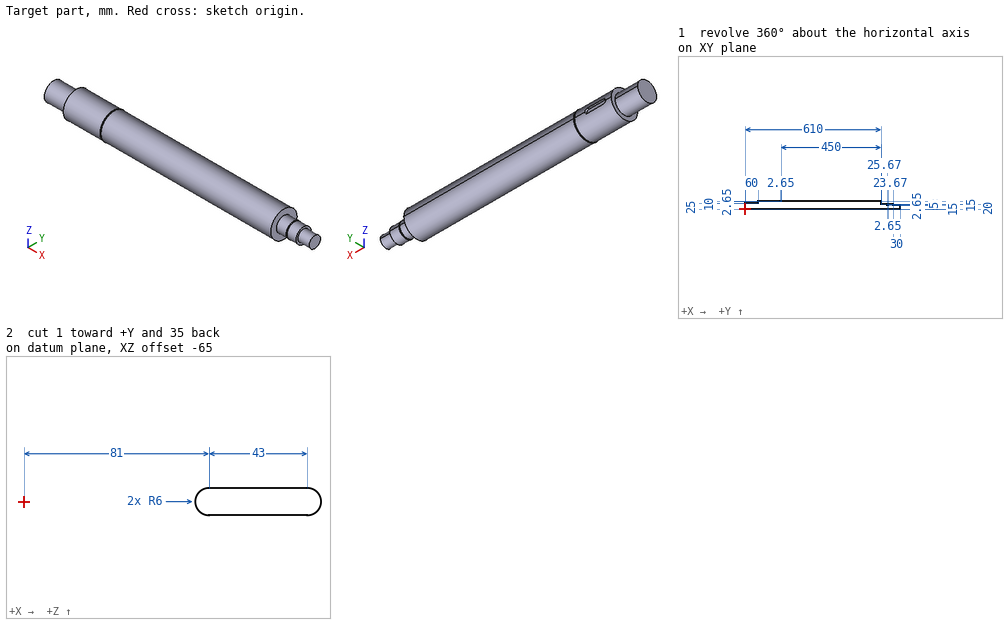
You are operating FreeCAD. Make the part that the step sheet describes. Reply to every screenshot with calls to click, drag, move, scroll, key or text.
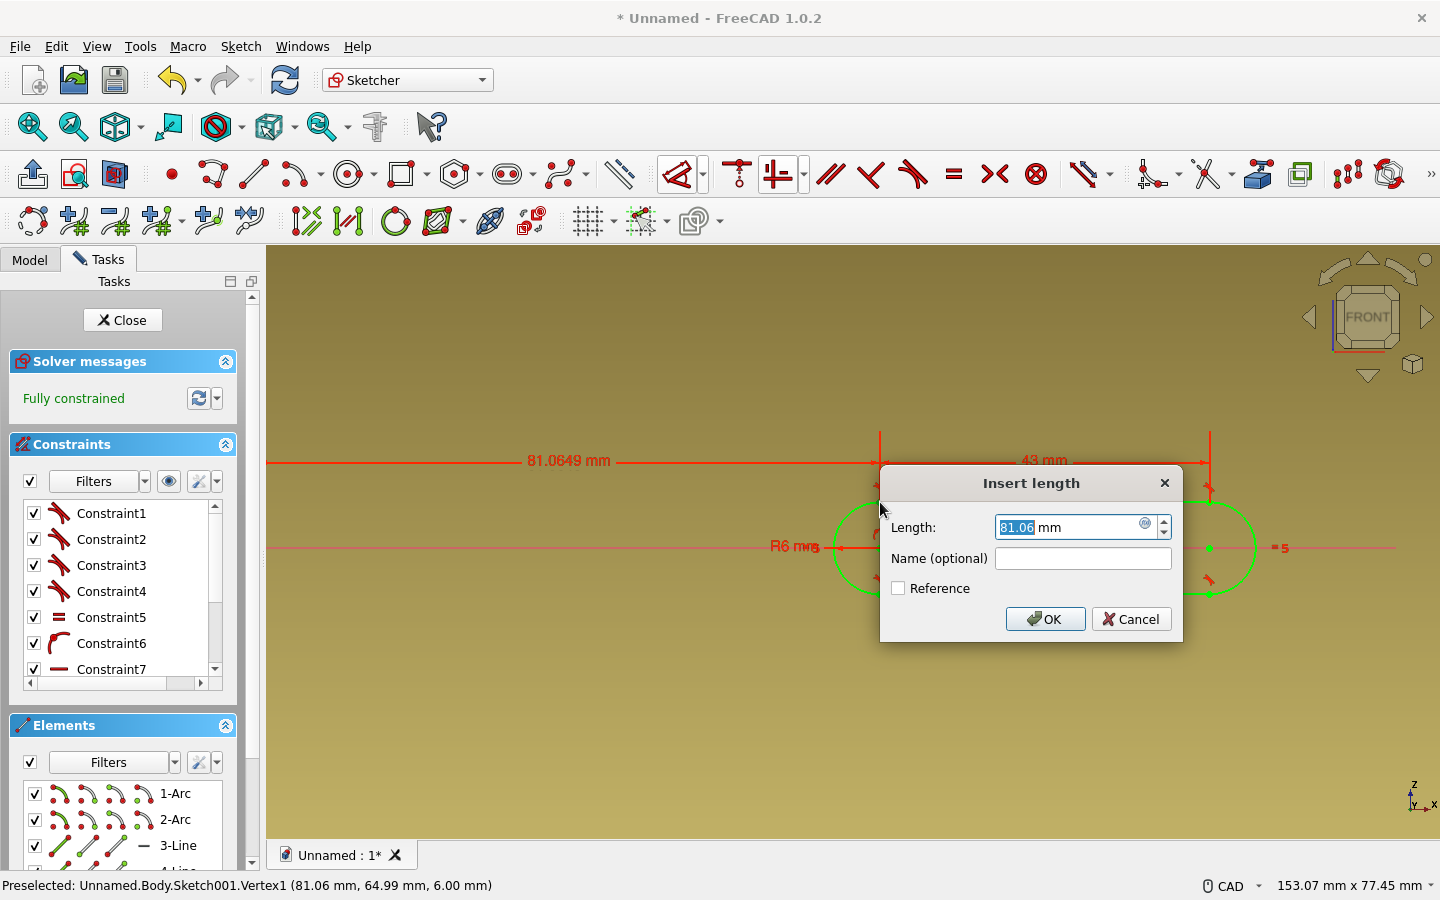
text(81)
key(Return)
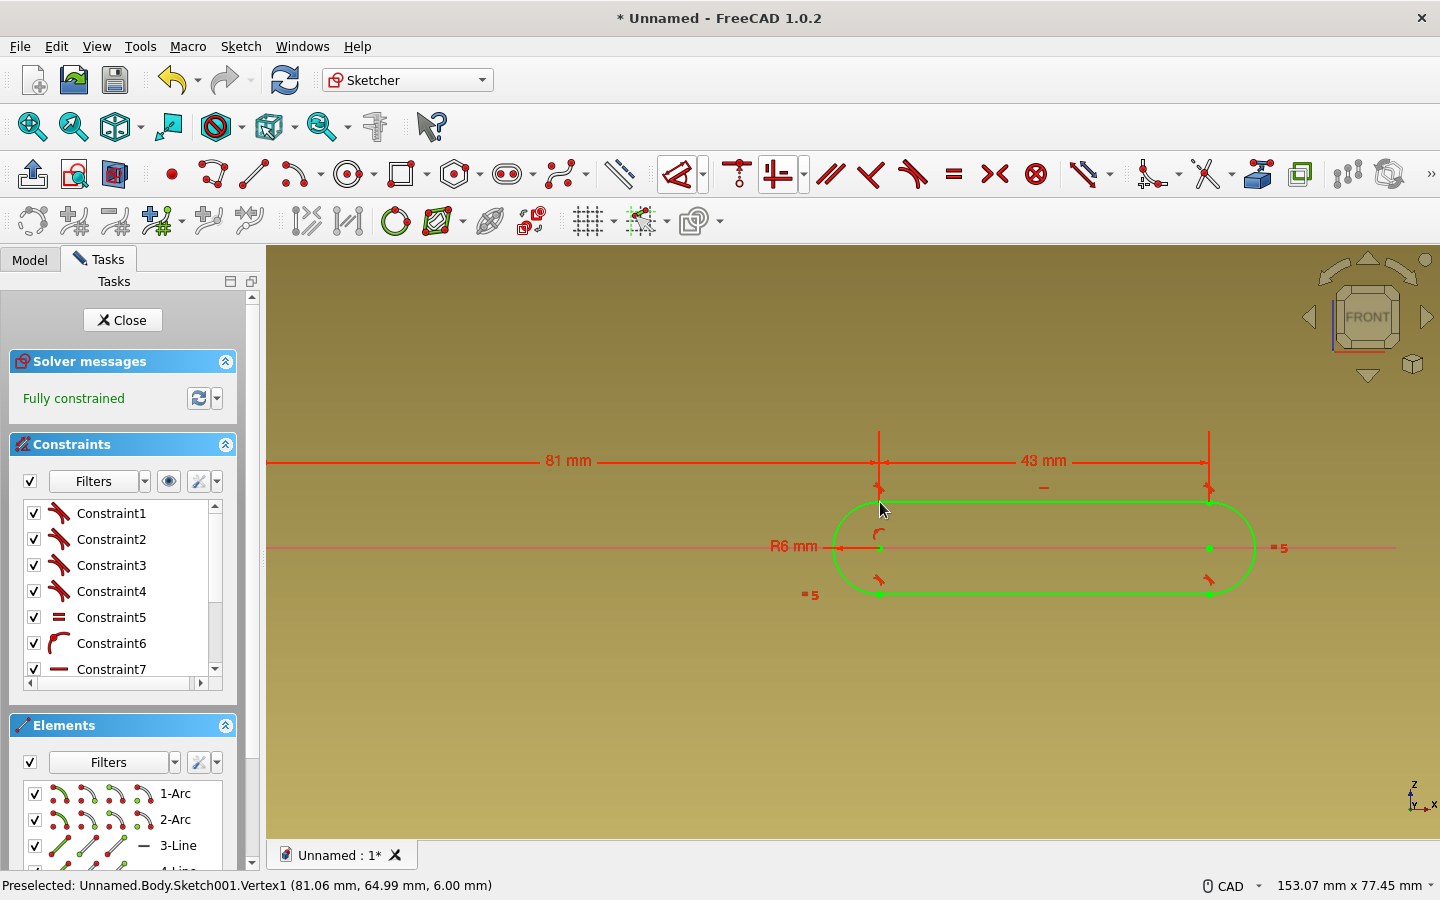
click(123, 320)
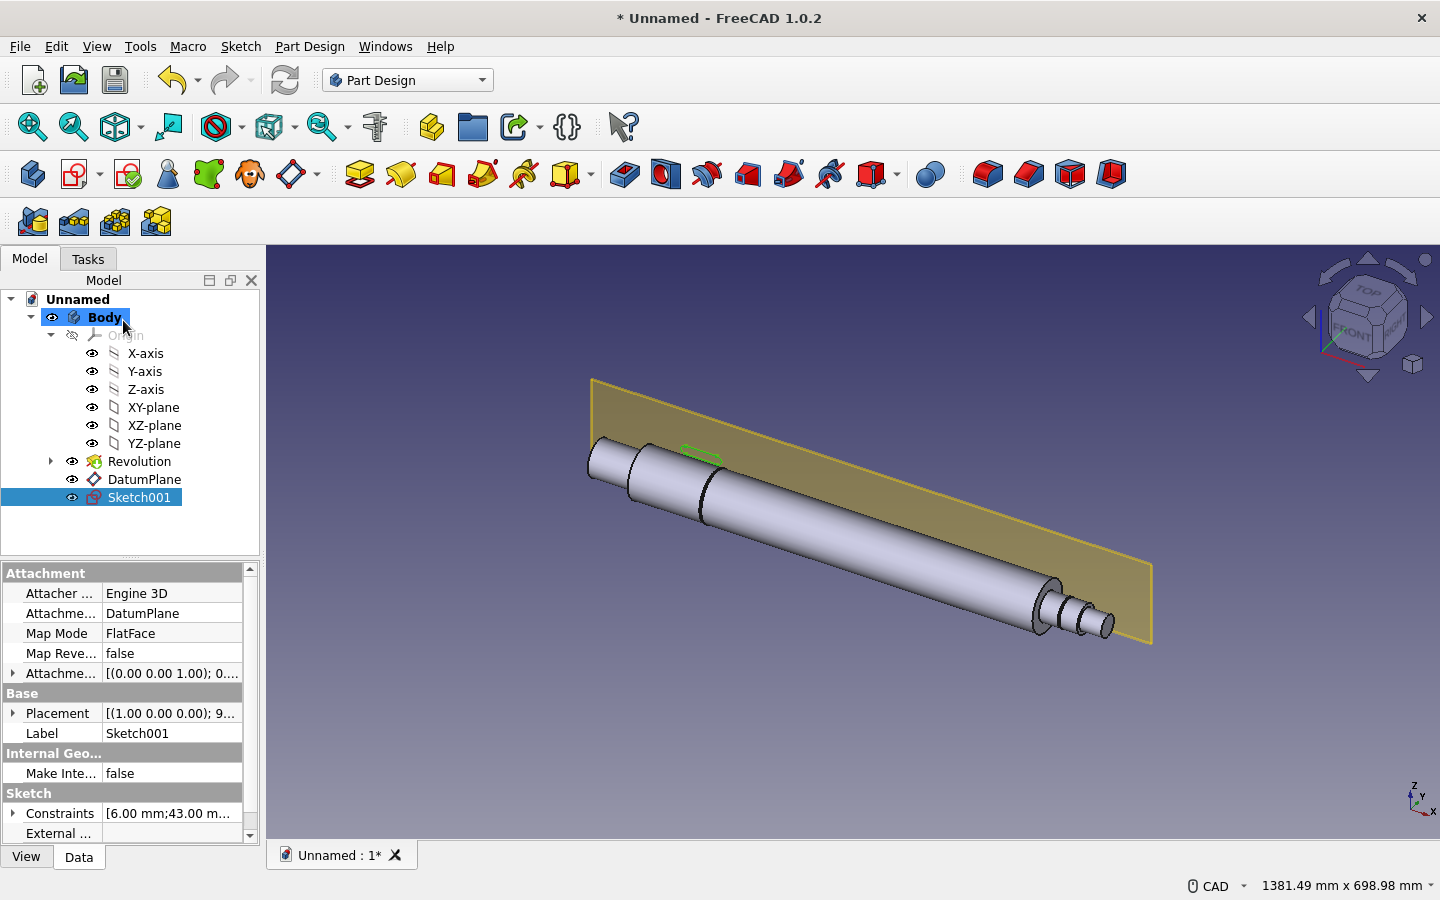
click(625, 174)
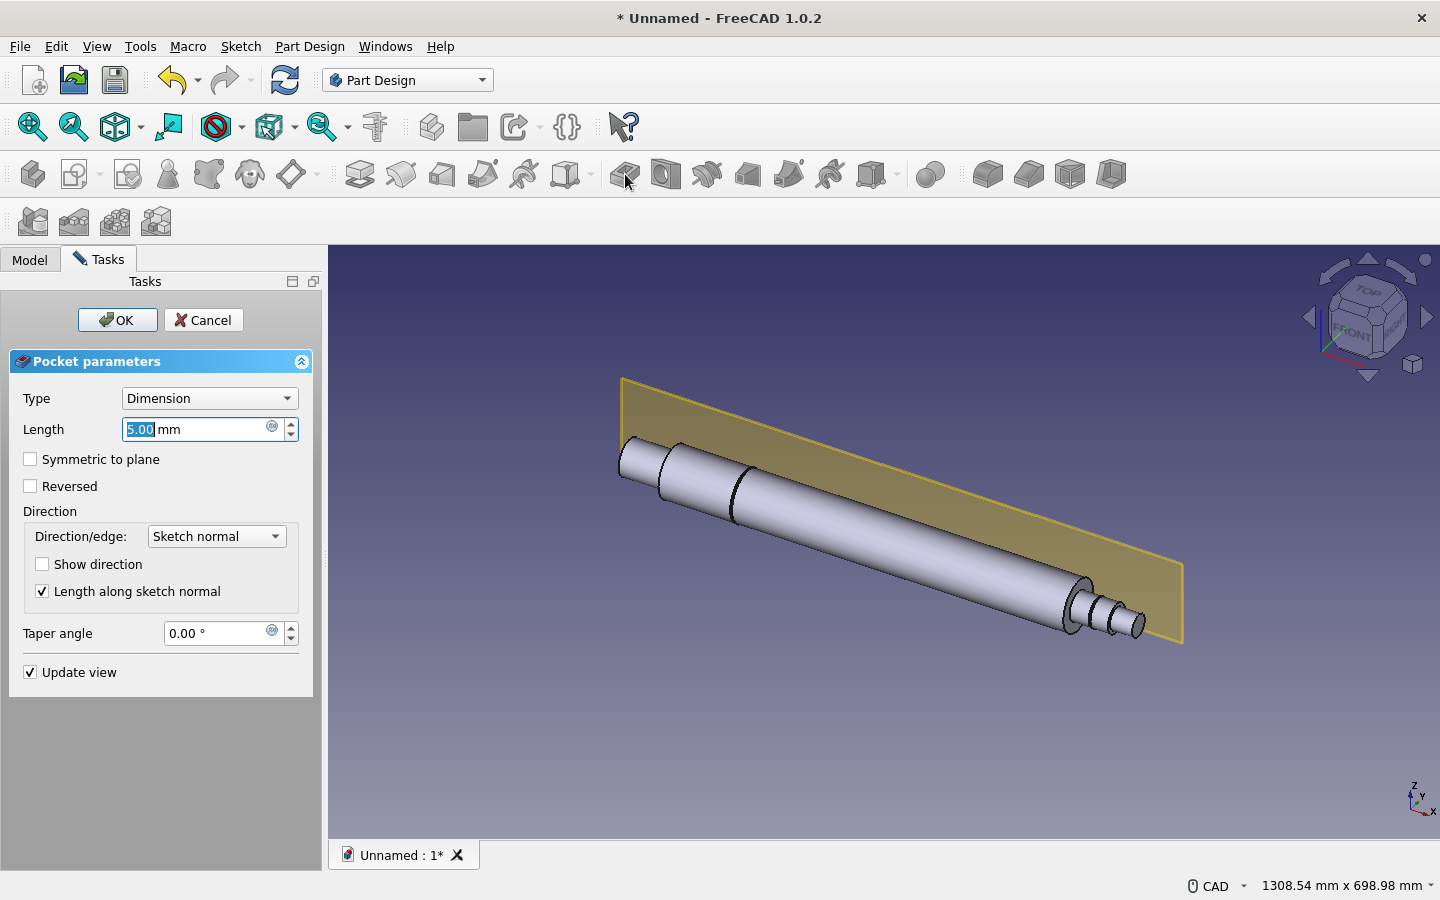
click(210, 398)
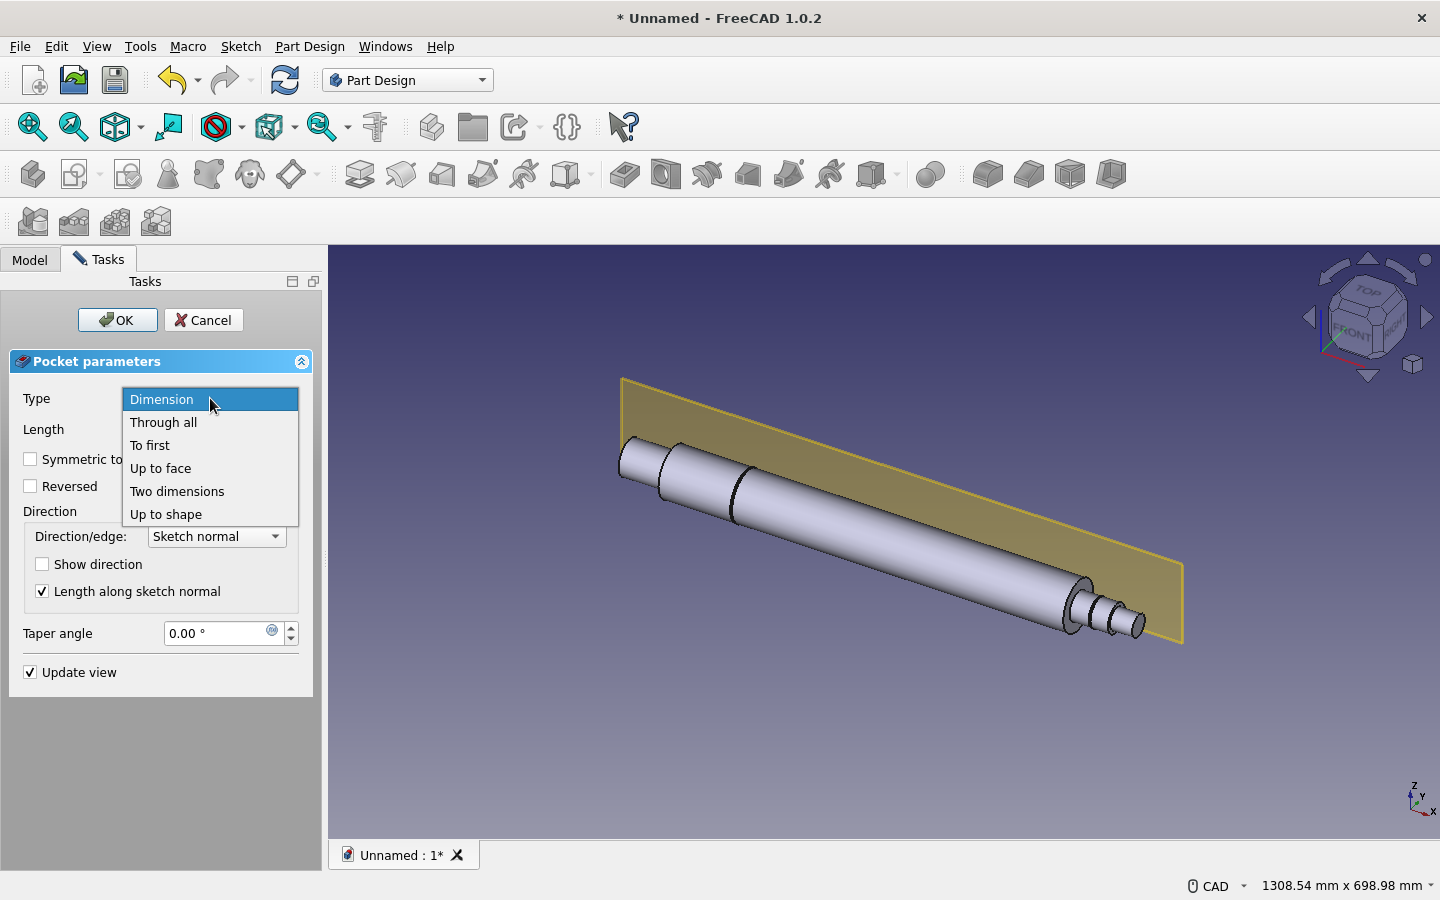
click(208, 492)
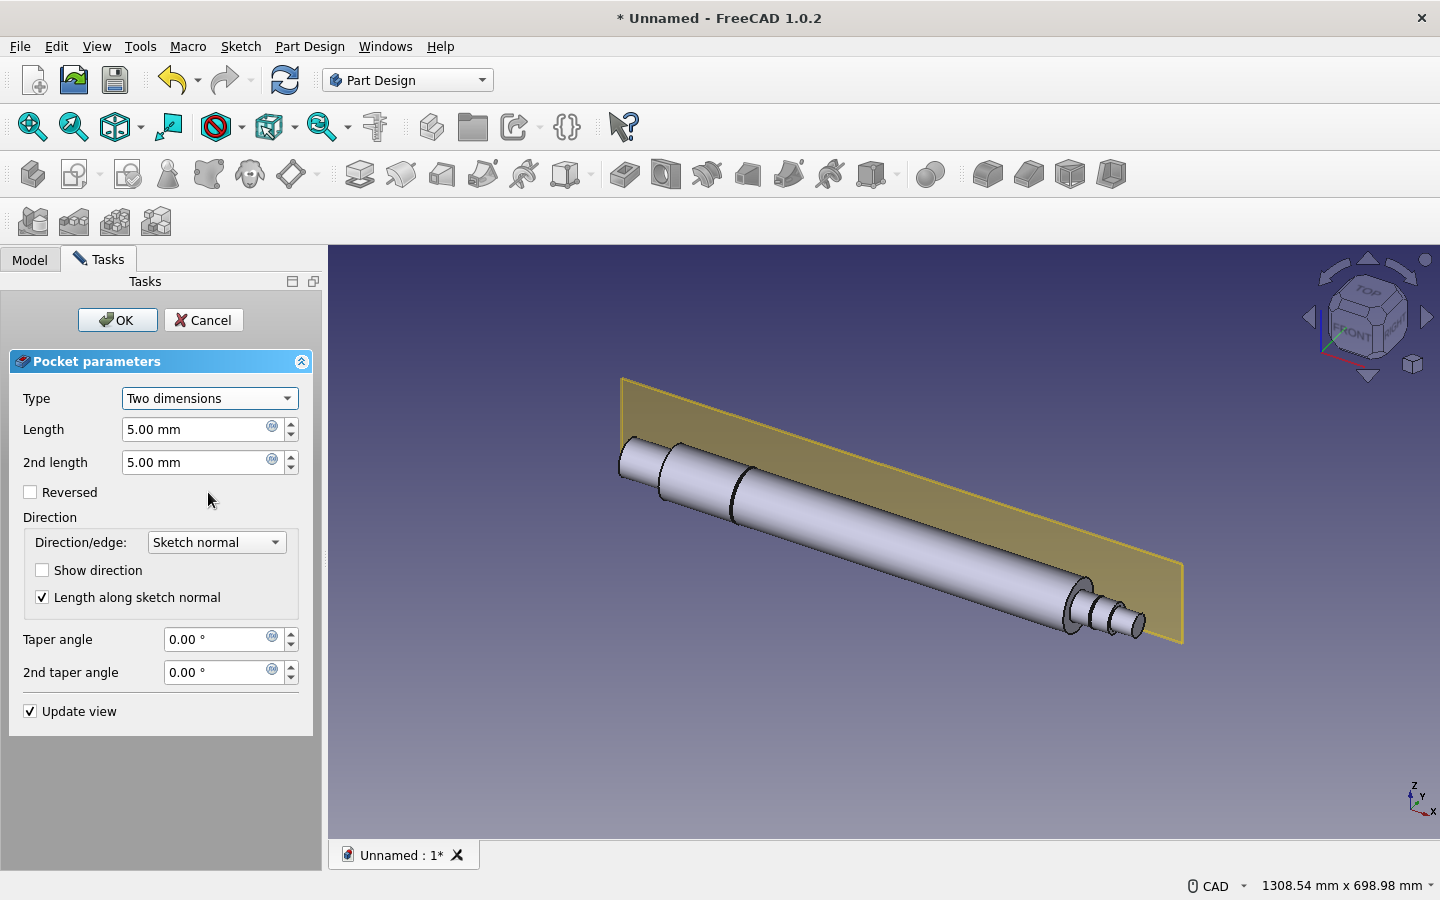
triple_click(204, 430)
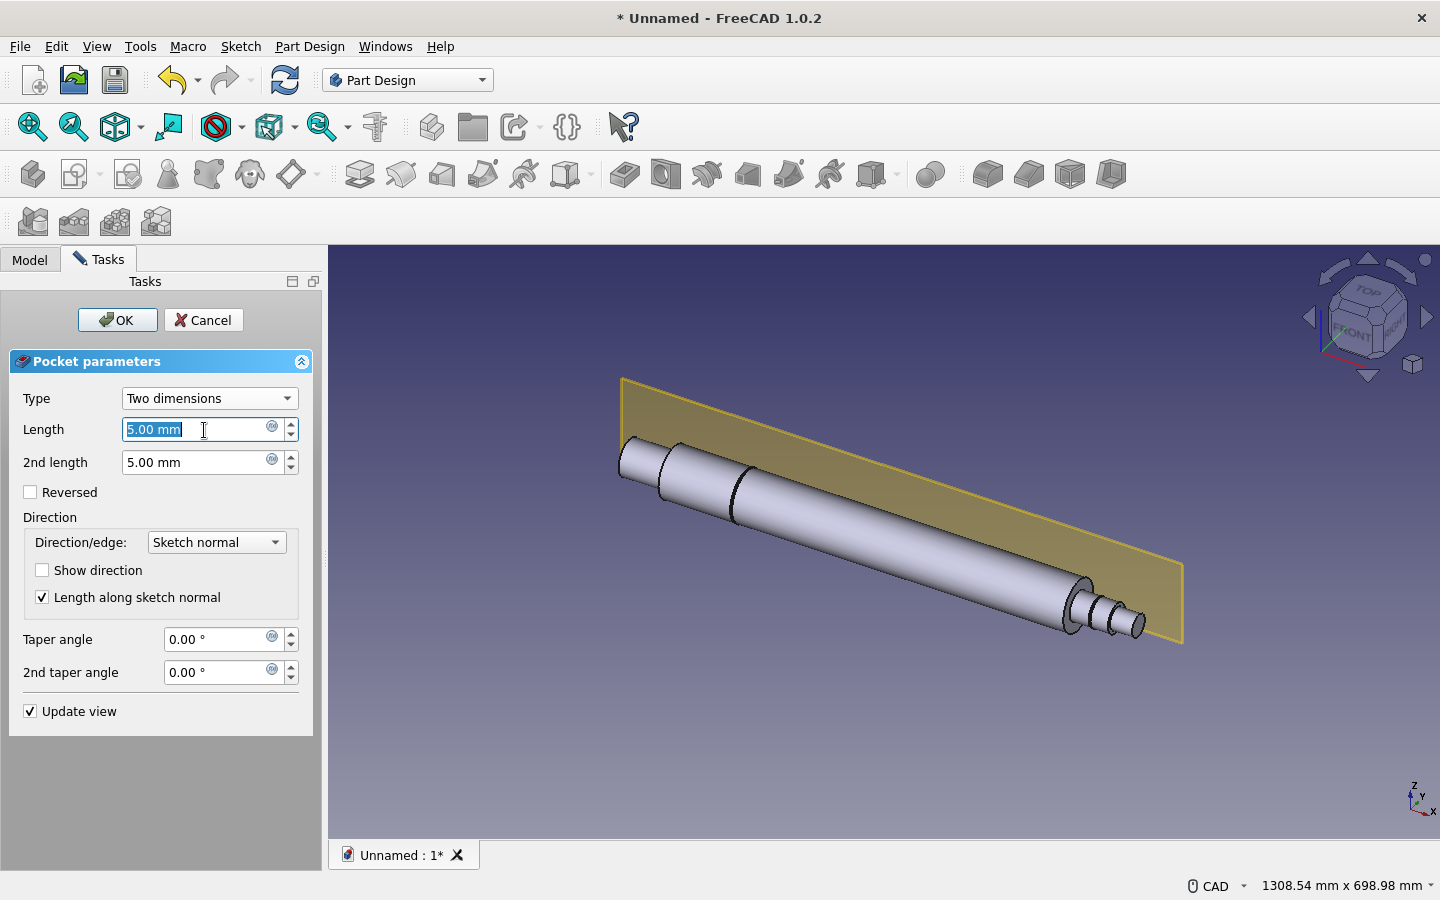
text(1)
key(Tab)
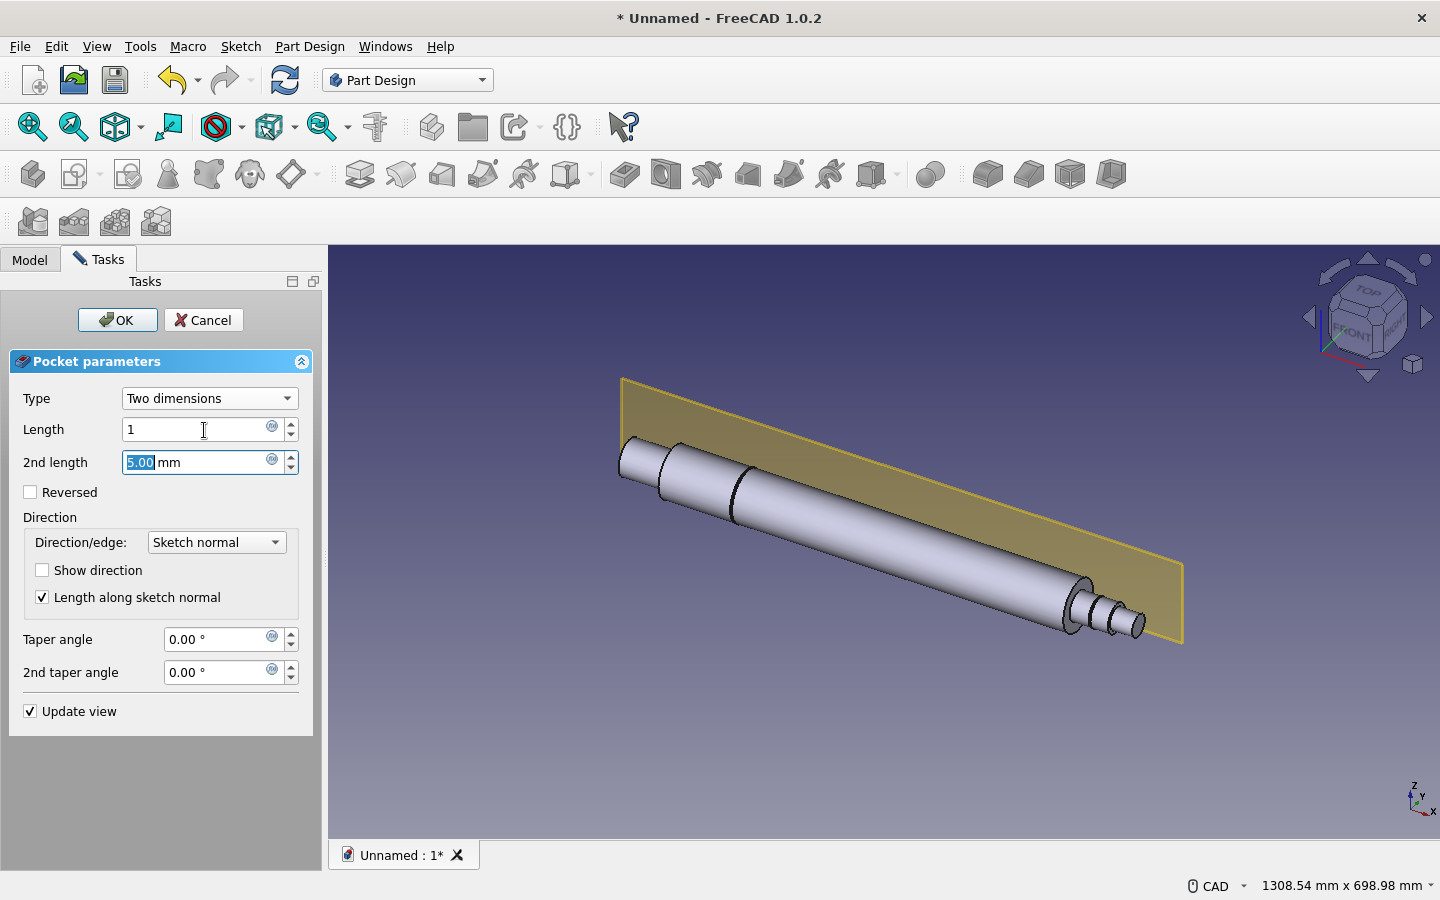
text(35)
key(Tab)